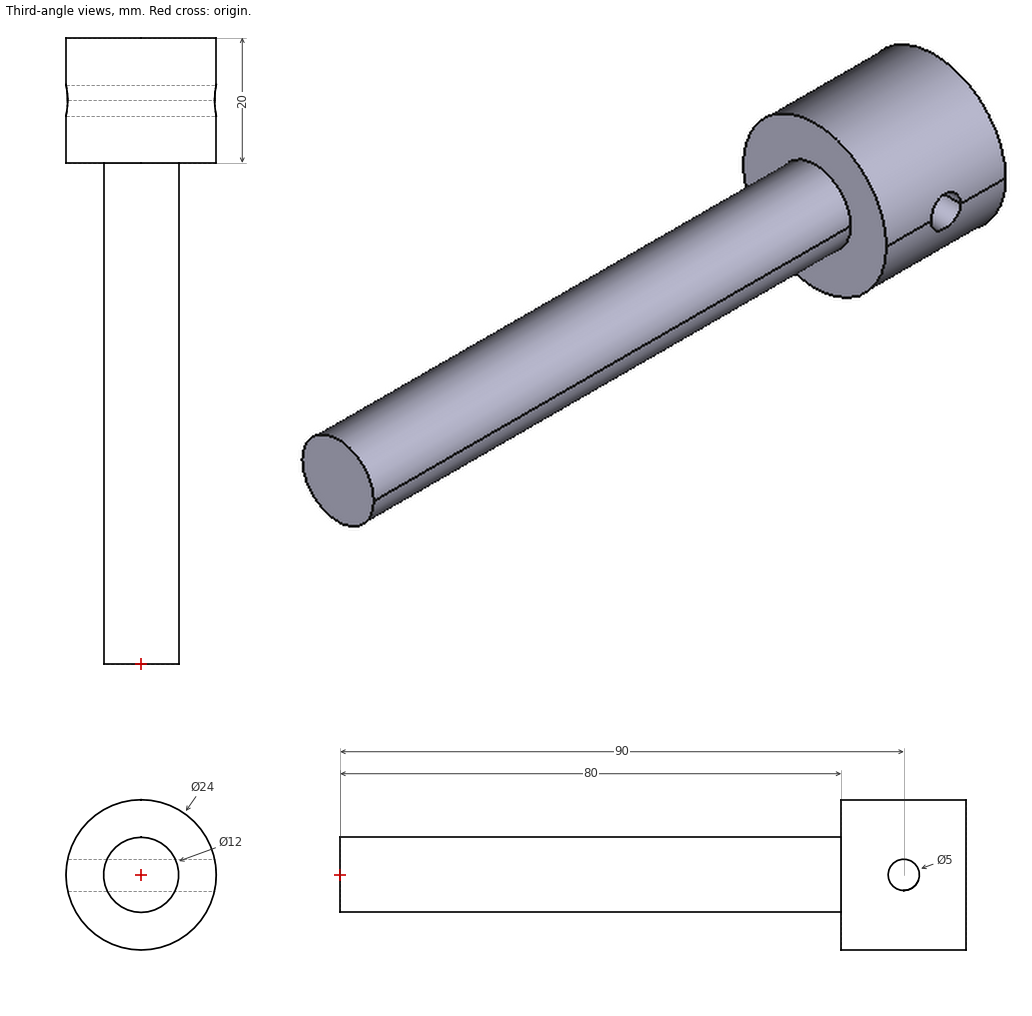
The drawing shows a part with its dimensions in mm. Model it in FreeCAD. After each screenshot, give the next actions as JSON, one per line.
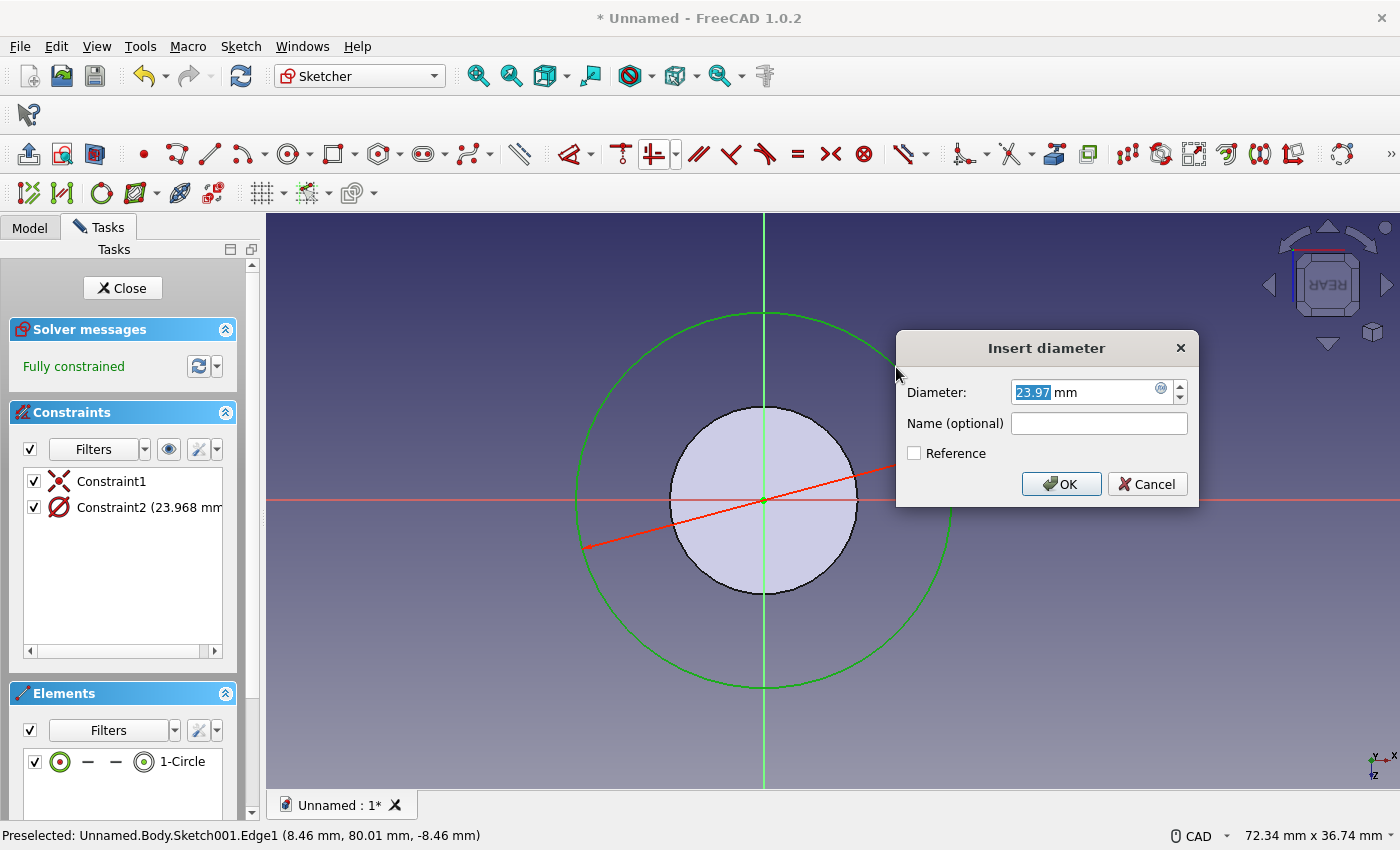
{"action": "type", "text": "24"}
{"action": "key", "text": "Return"}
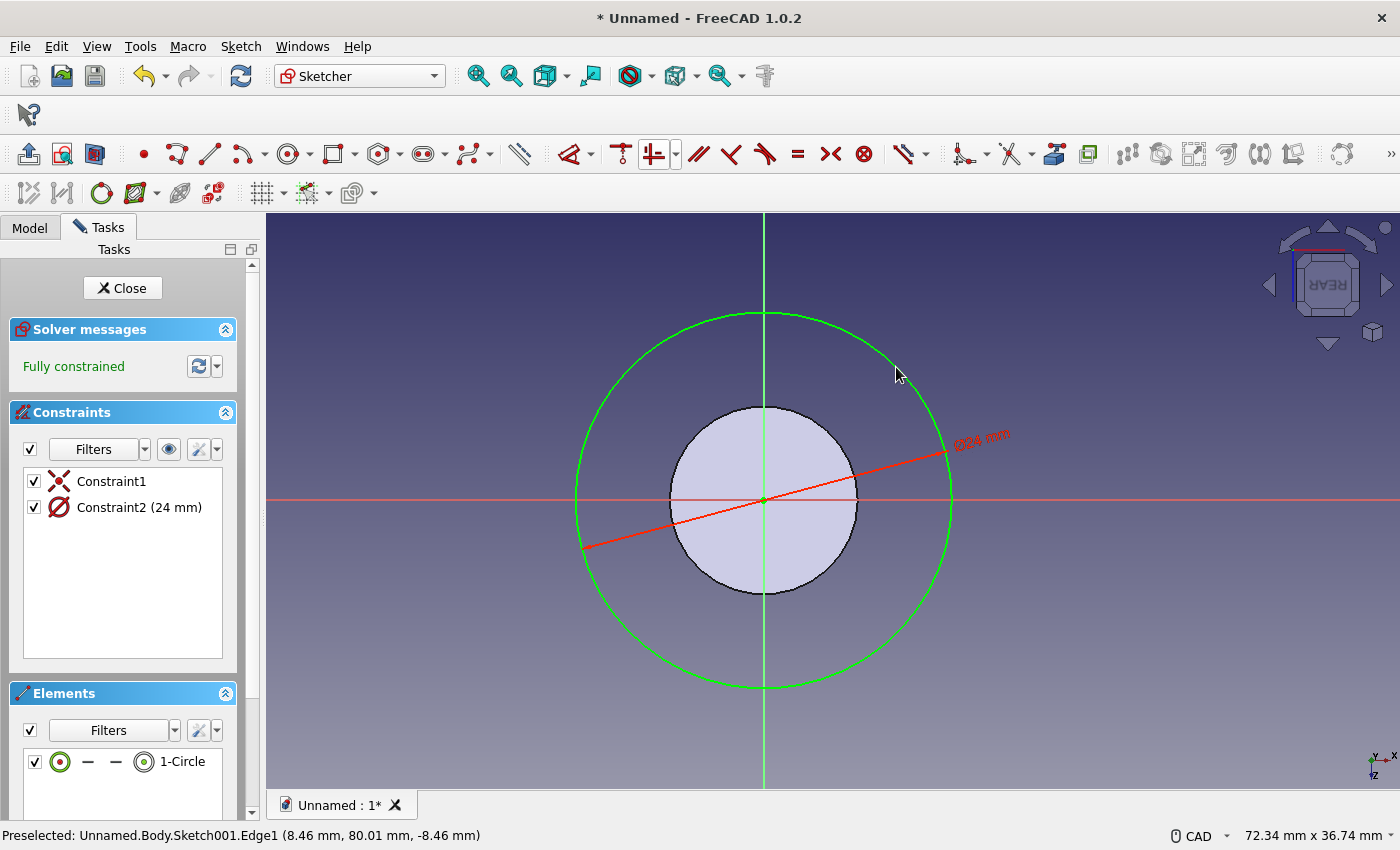
{"action": "left_click", "coordinate": [123, 288]}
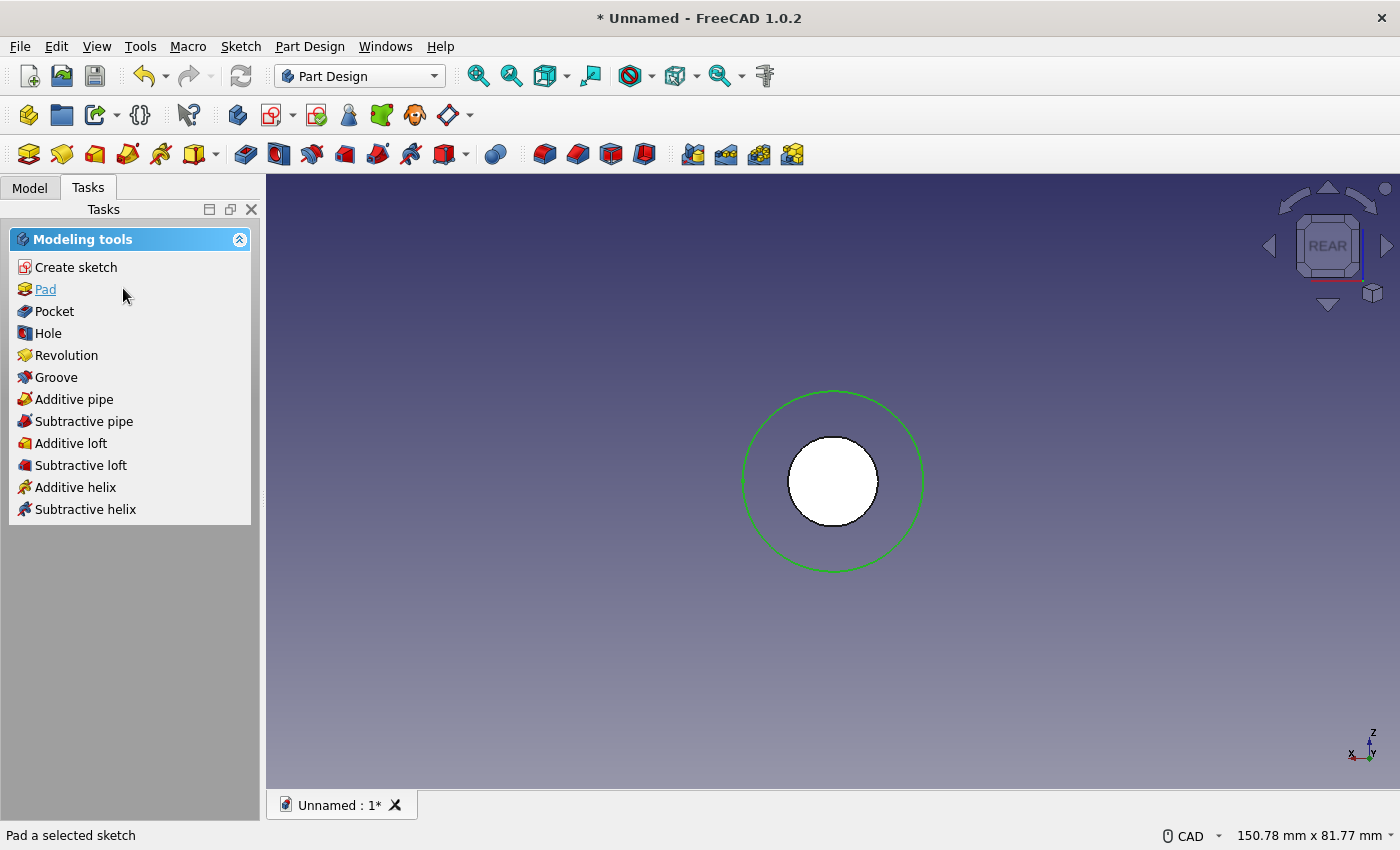
{"action": "left_click", "coordinate": [29, 154]}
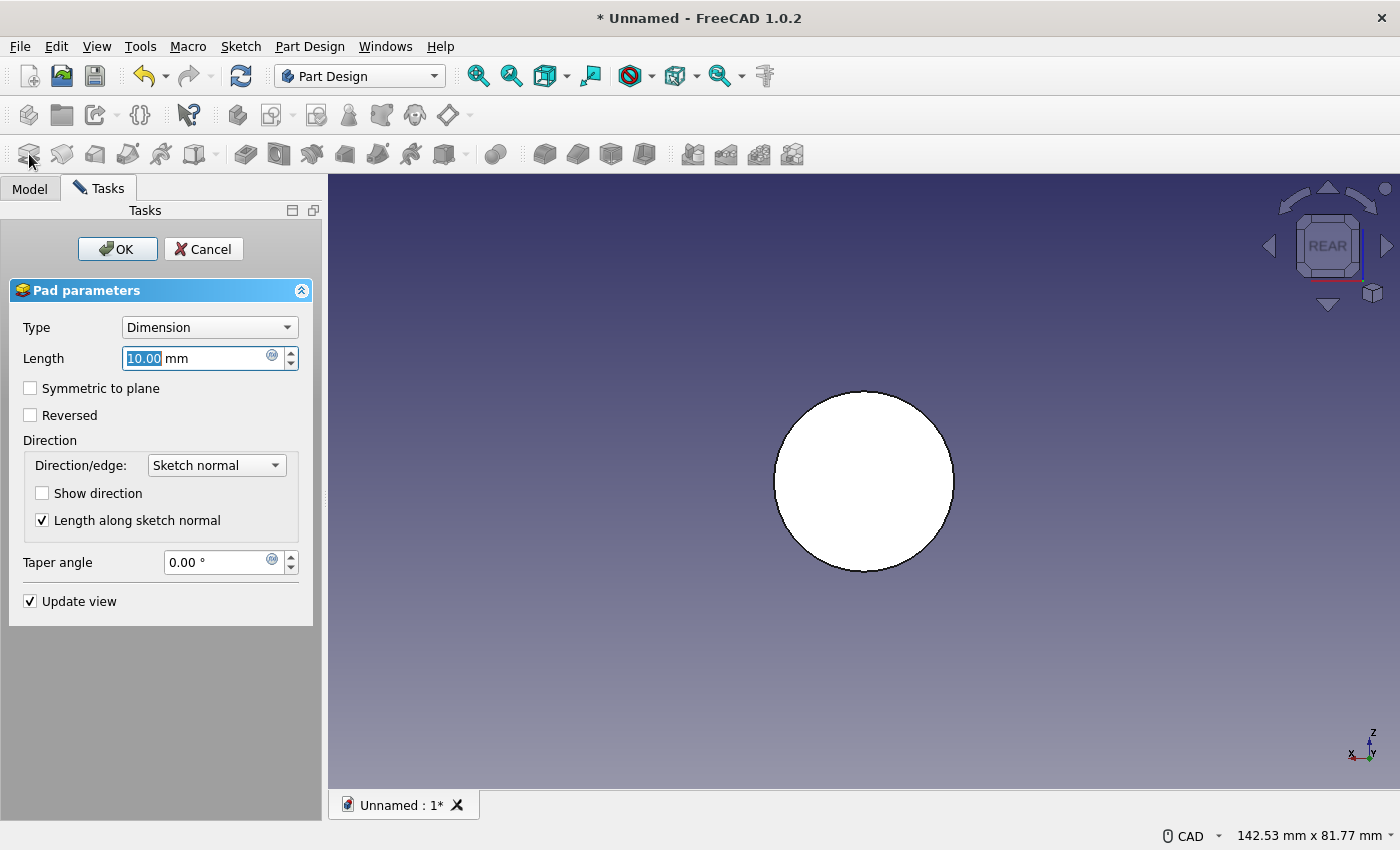
{"action": "type", "text": "20"}
{"action": "key", "text": "Tab"}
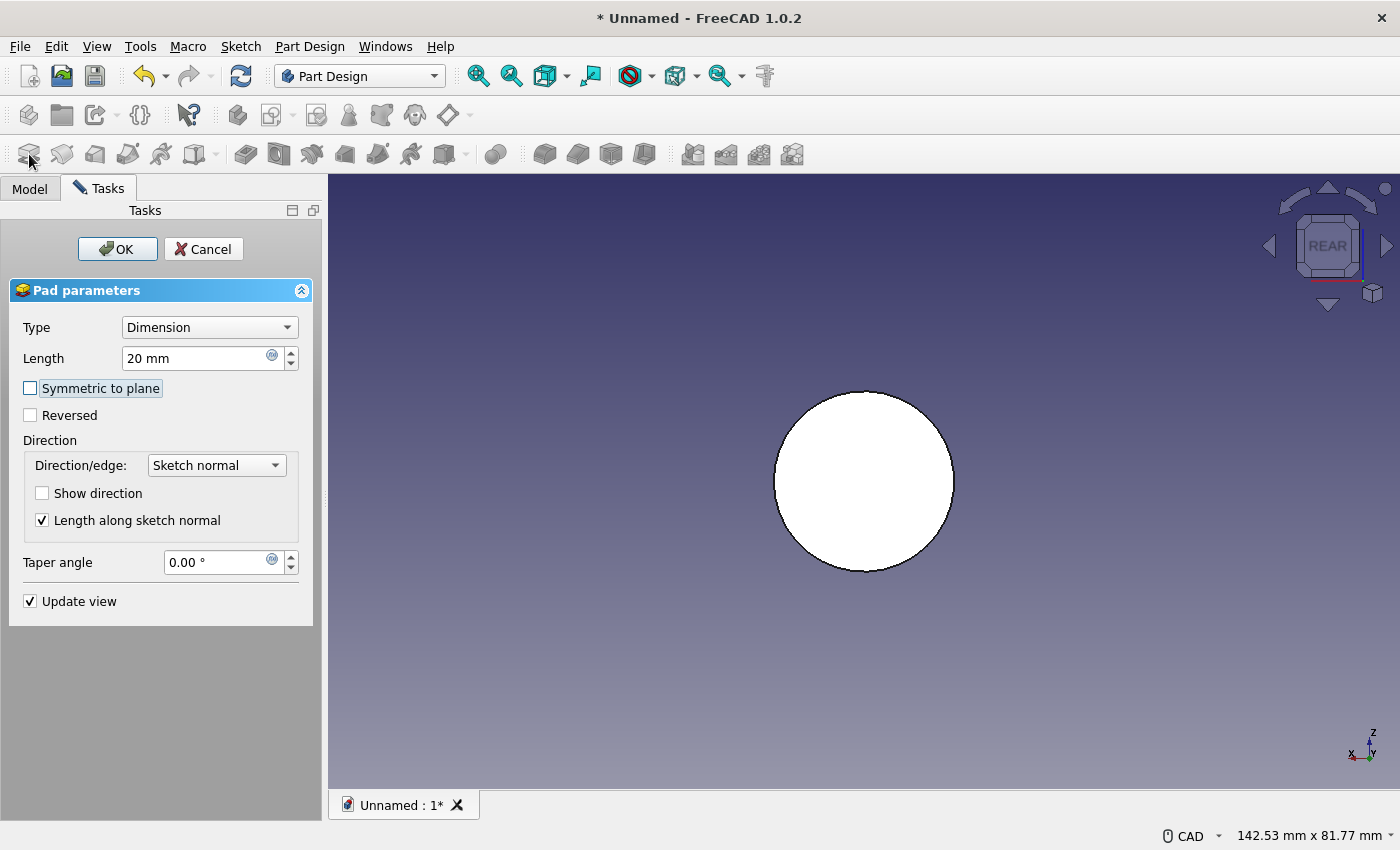
{"action": "left_click", "coordinate": [118, 249]}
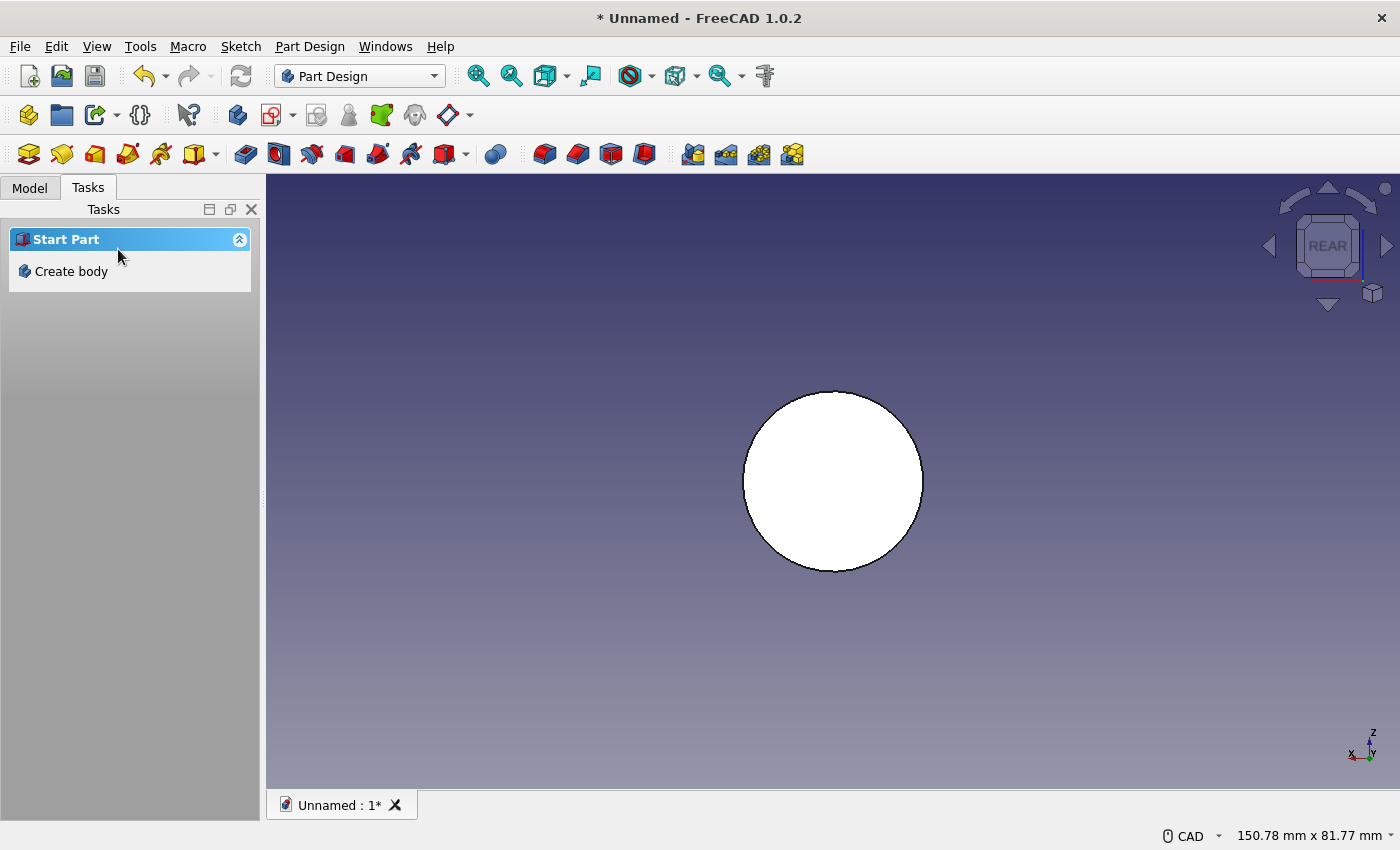
{"action": "key", "text": "v f"}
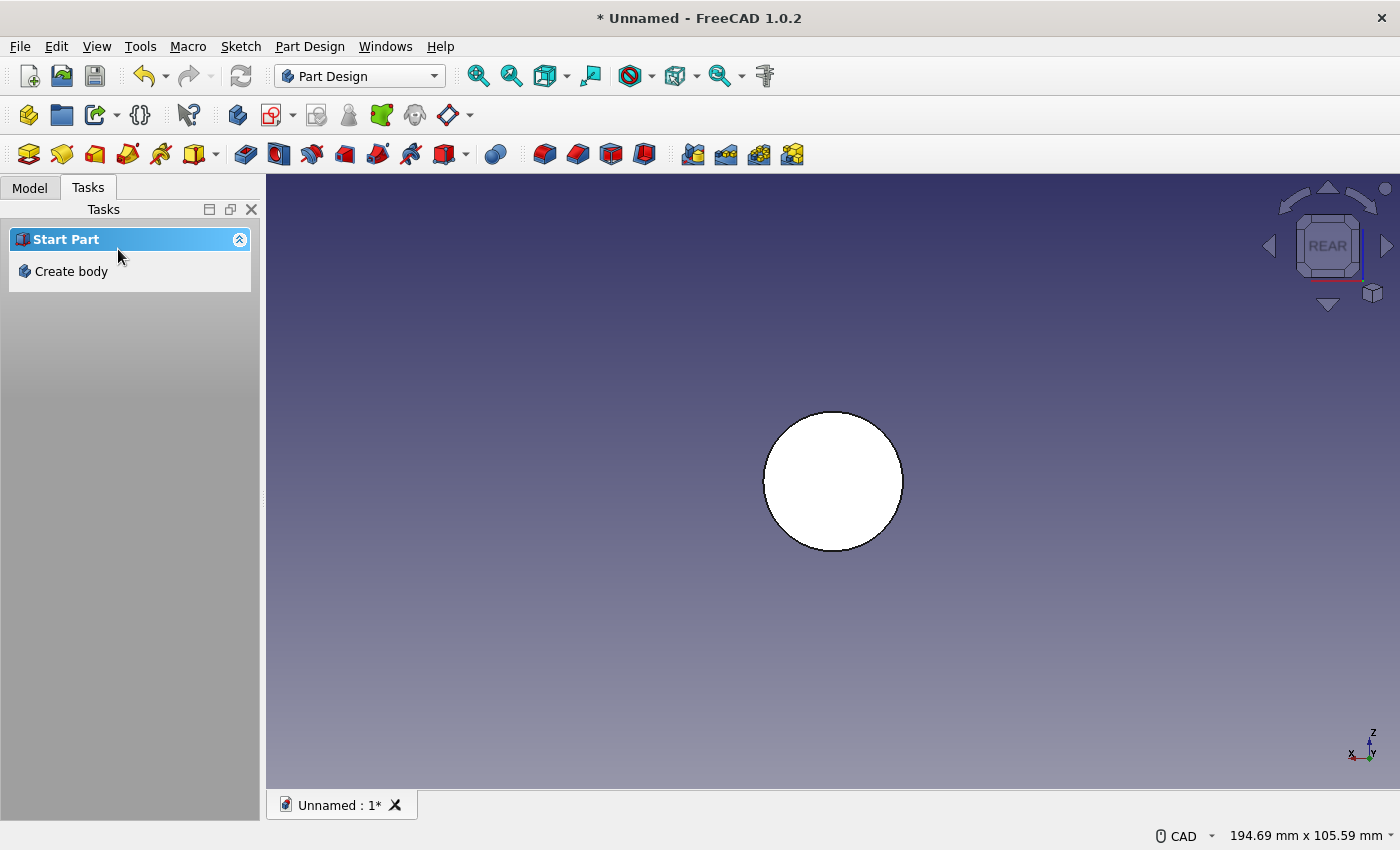
{"action": "left_click", "coordinate": [270, 116]}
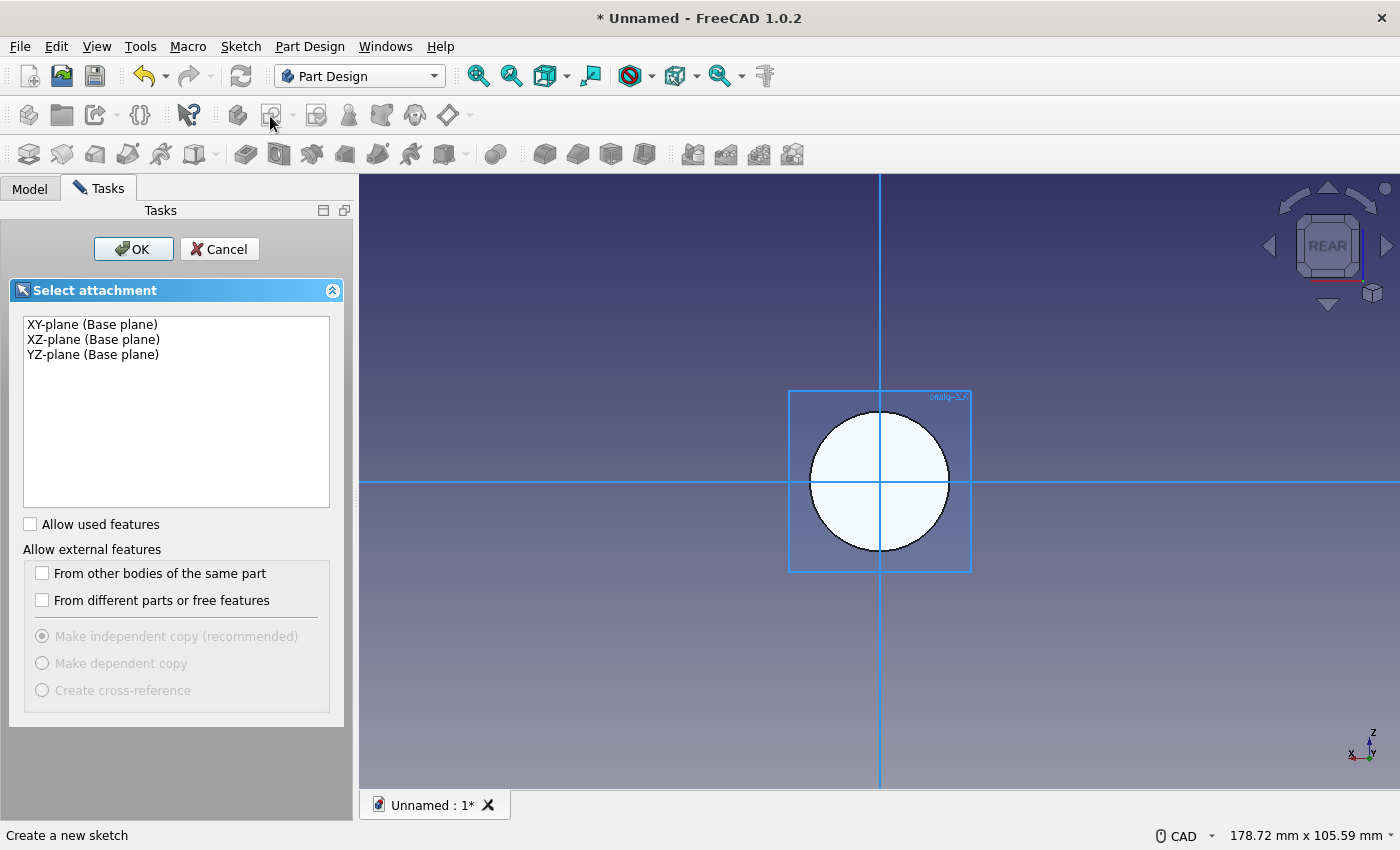
{"action": "left_click", "coordinate": [84, 354]}